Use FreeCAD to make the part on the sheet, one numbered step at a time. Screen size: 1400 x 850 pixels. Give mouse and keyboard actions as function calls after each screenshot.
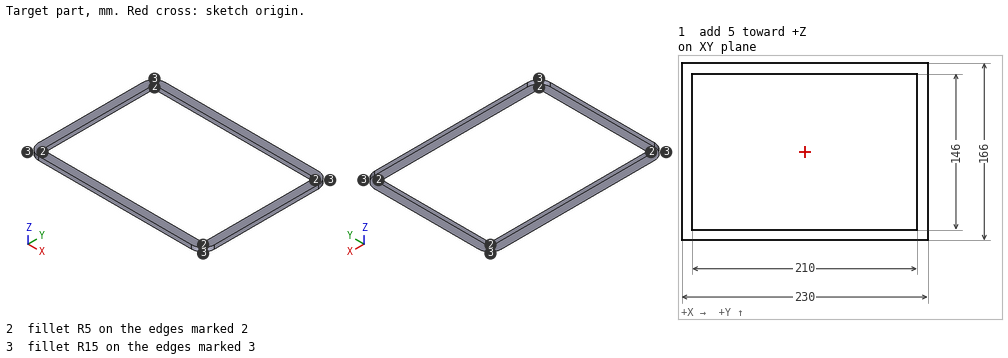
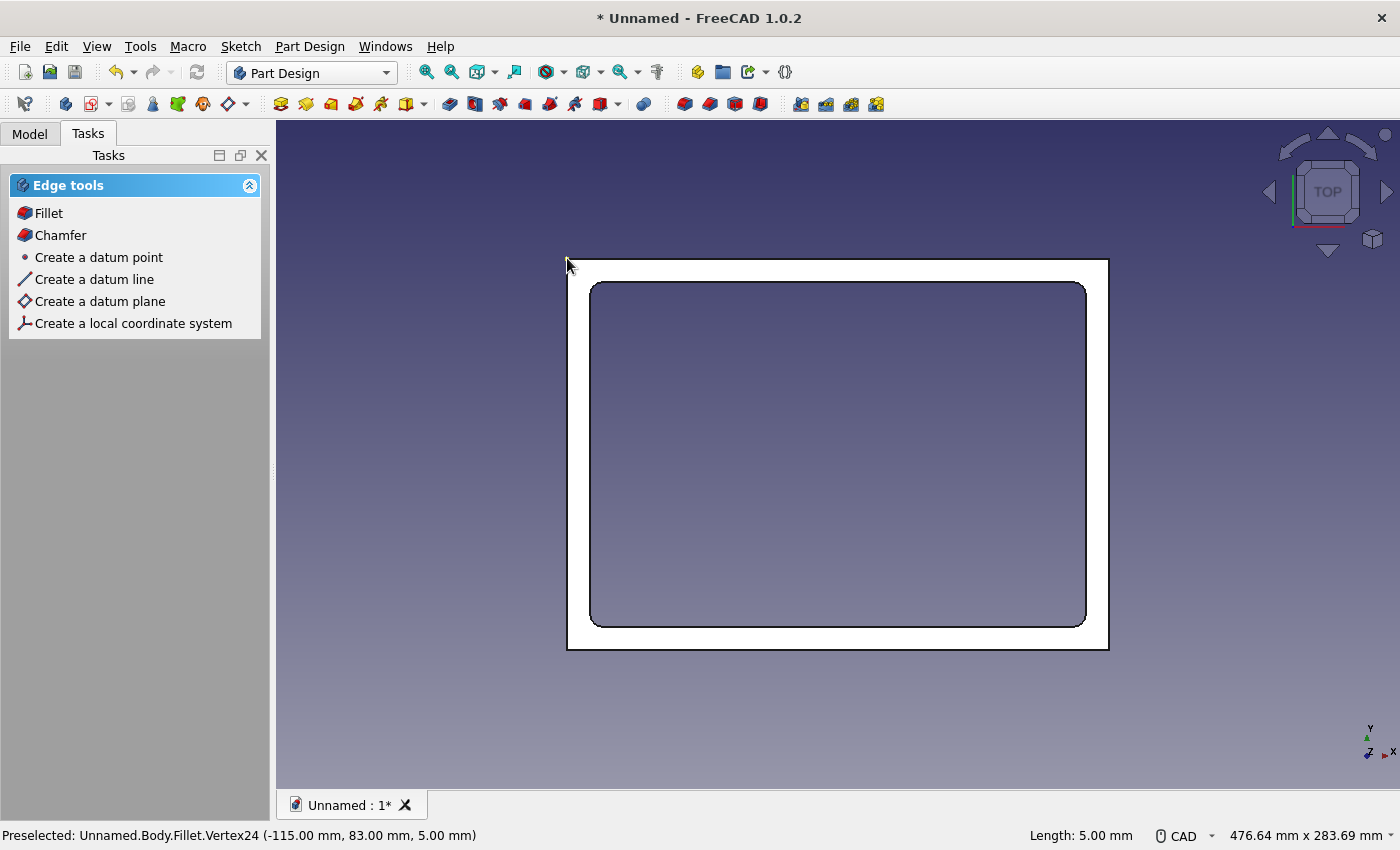
key(0)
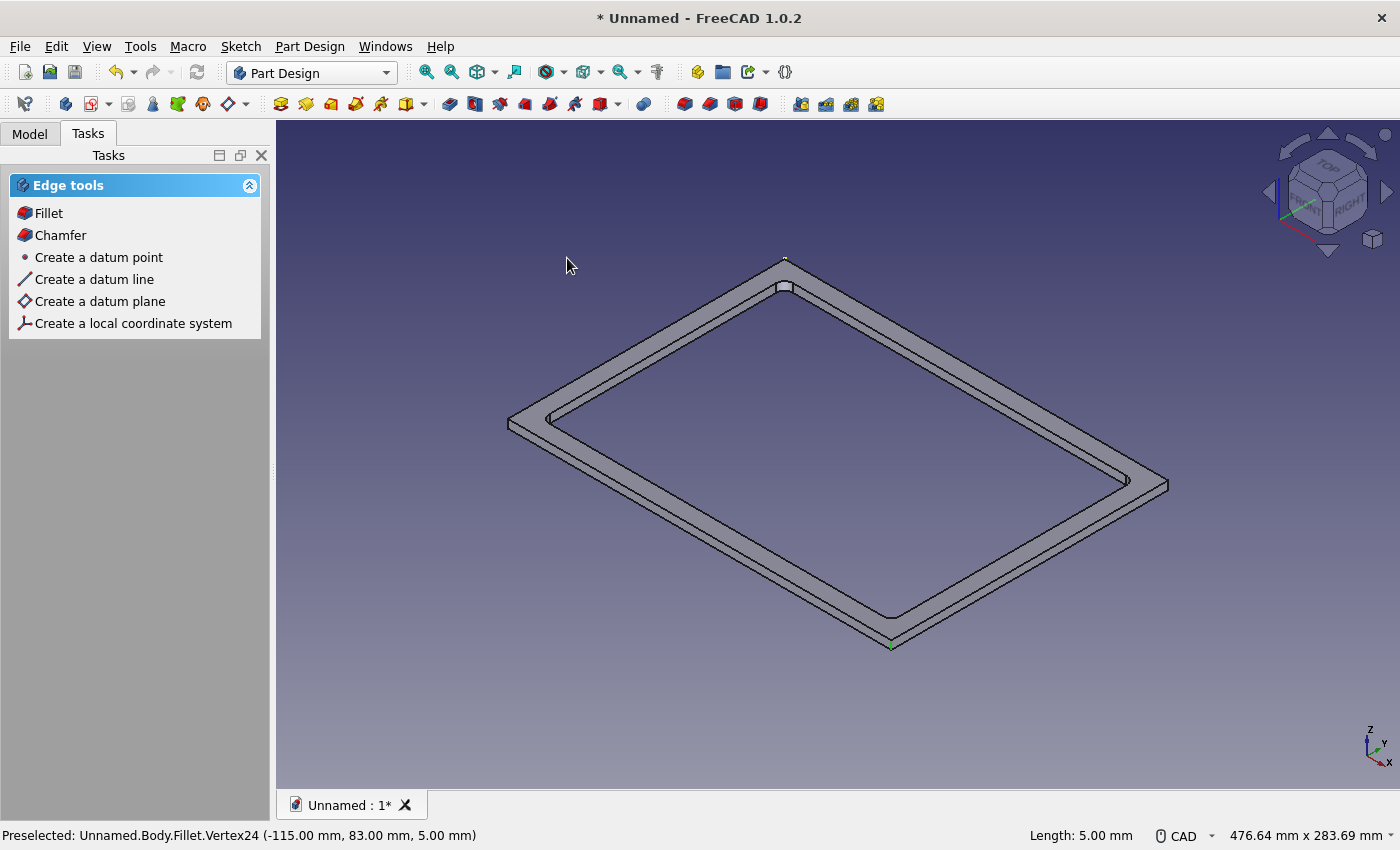
scroll(785, 263, up, 7)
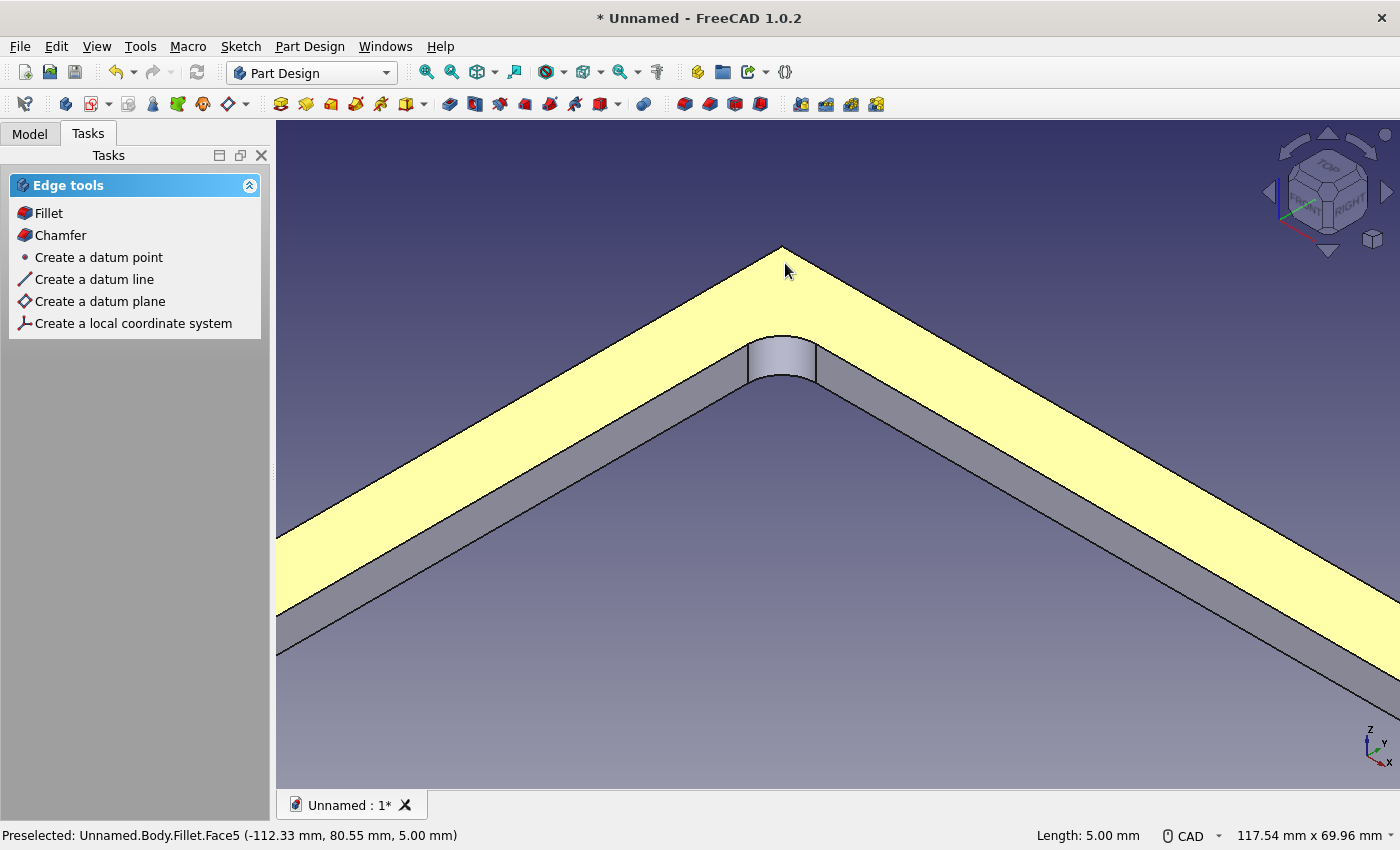
key(v)
key(f)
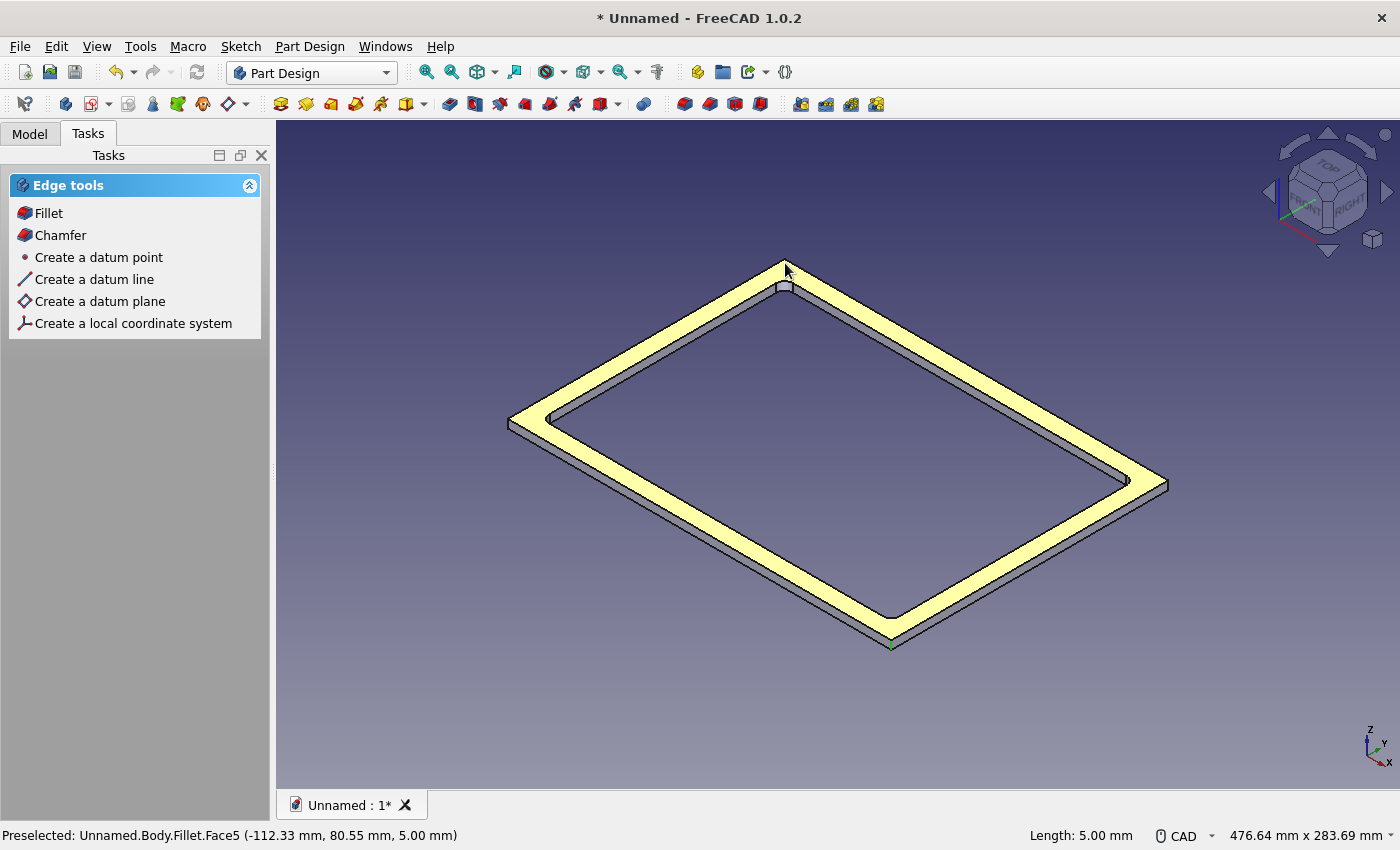
key(1)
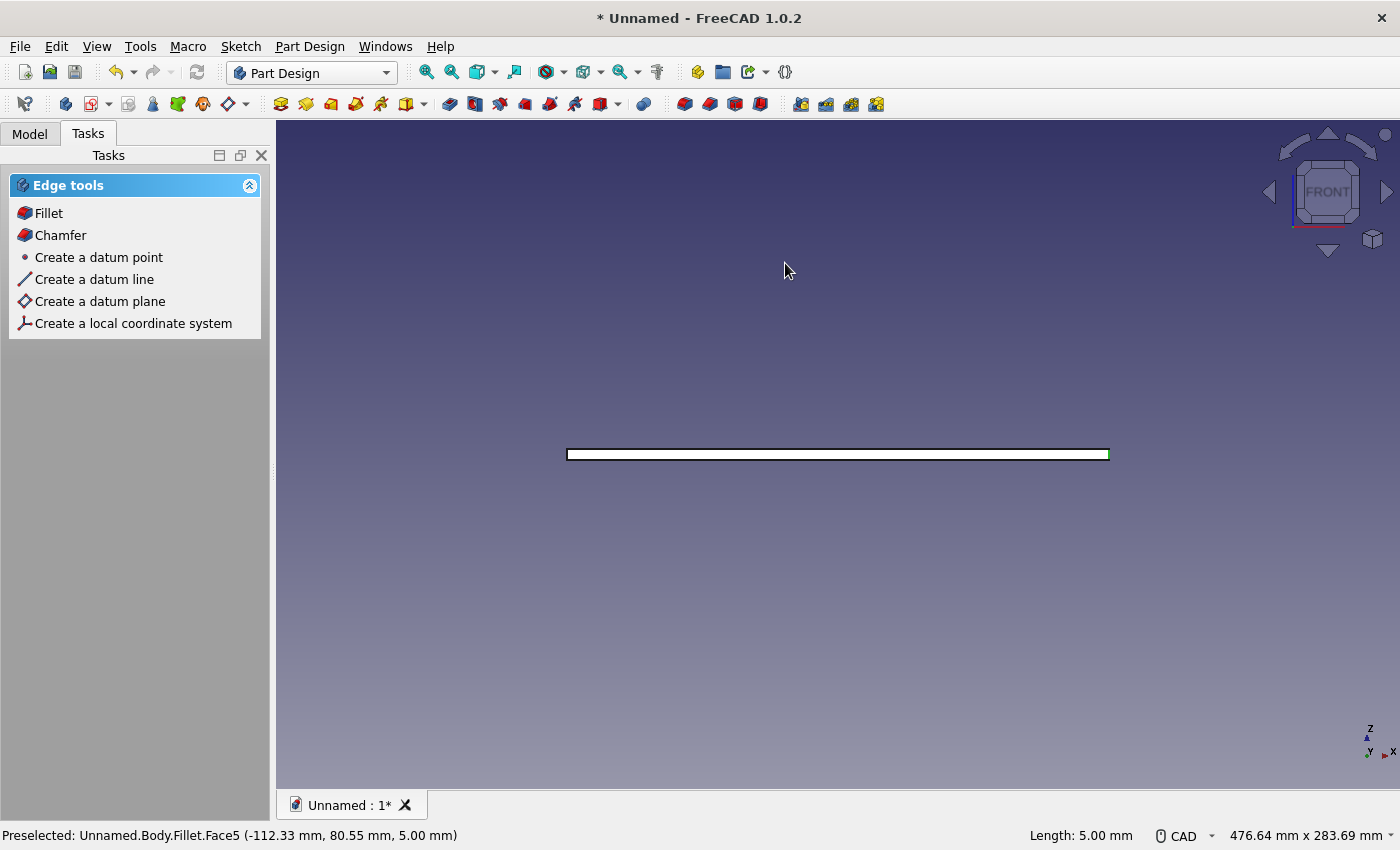
scroll(567, 453, up, 7)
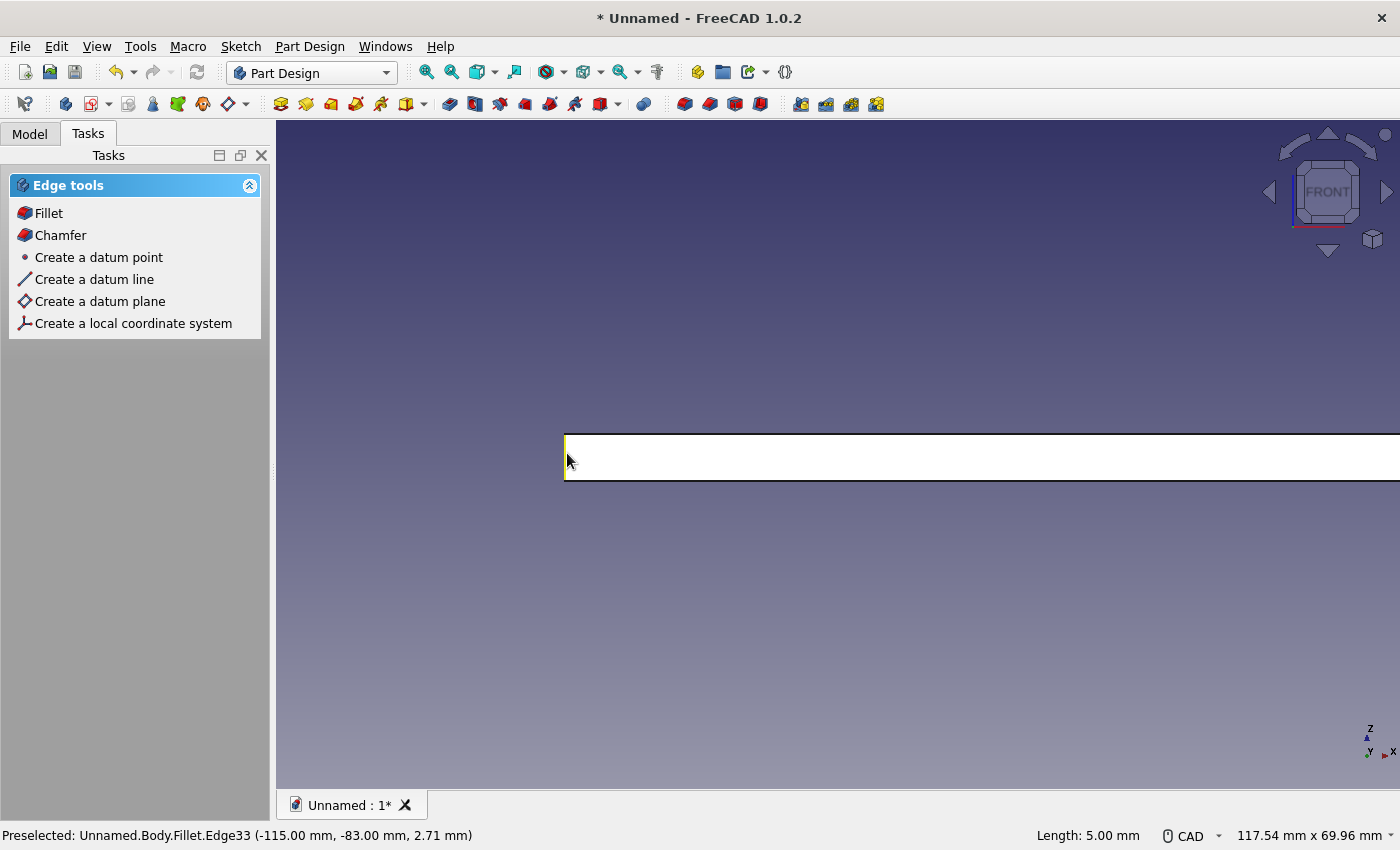
click(565, 457, ctrl)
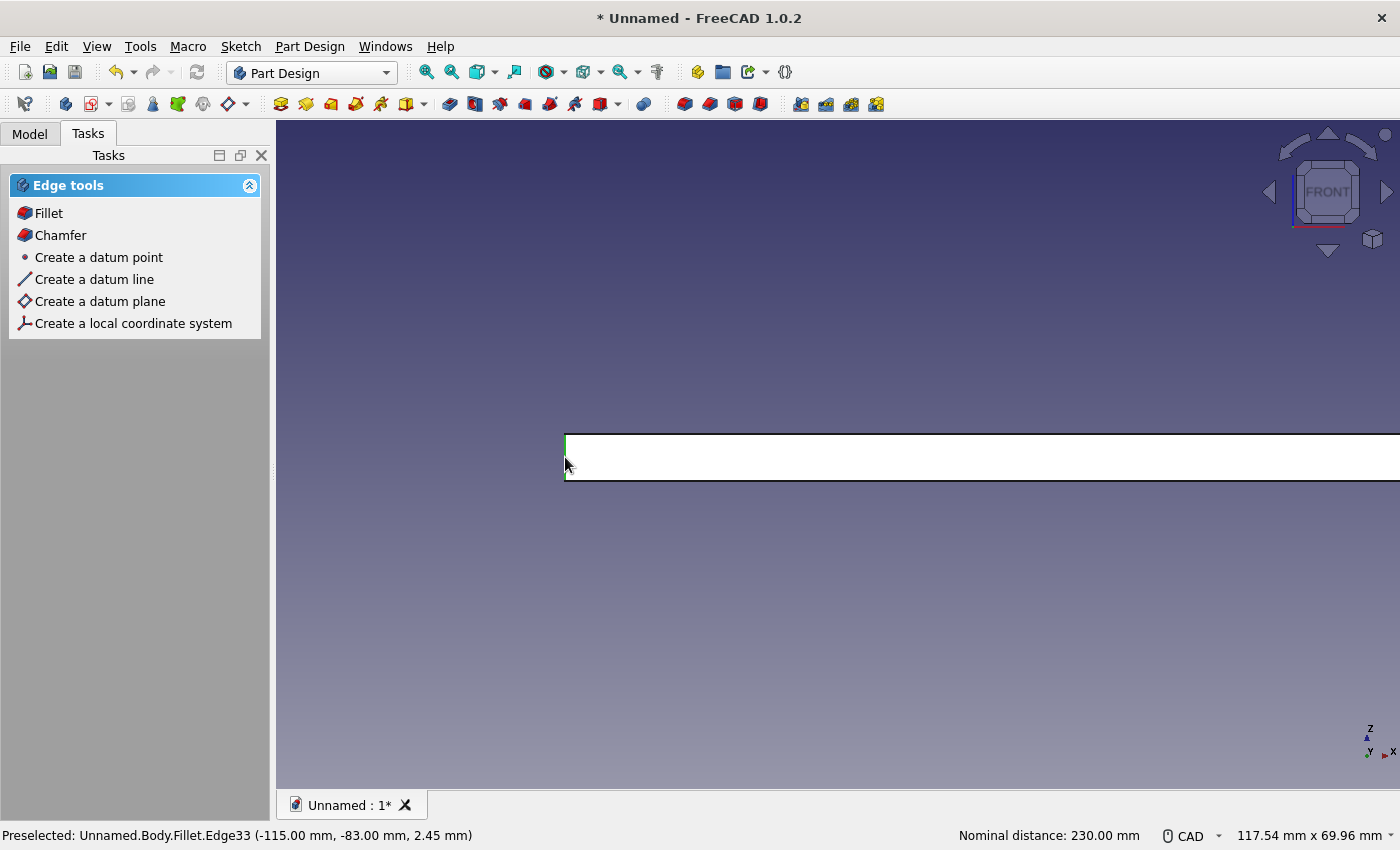
key(v)
key(f)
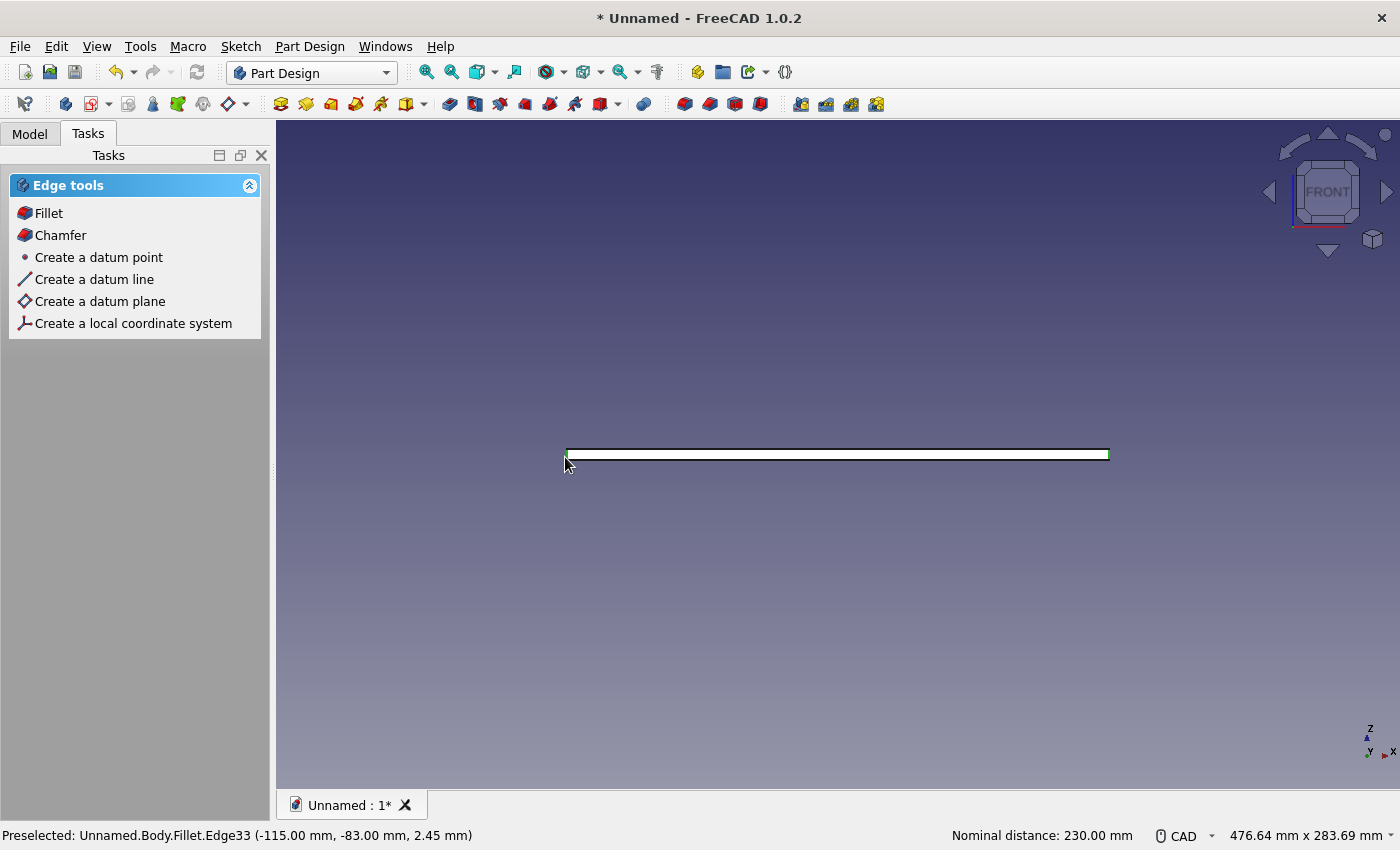
key(3)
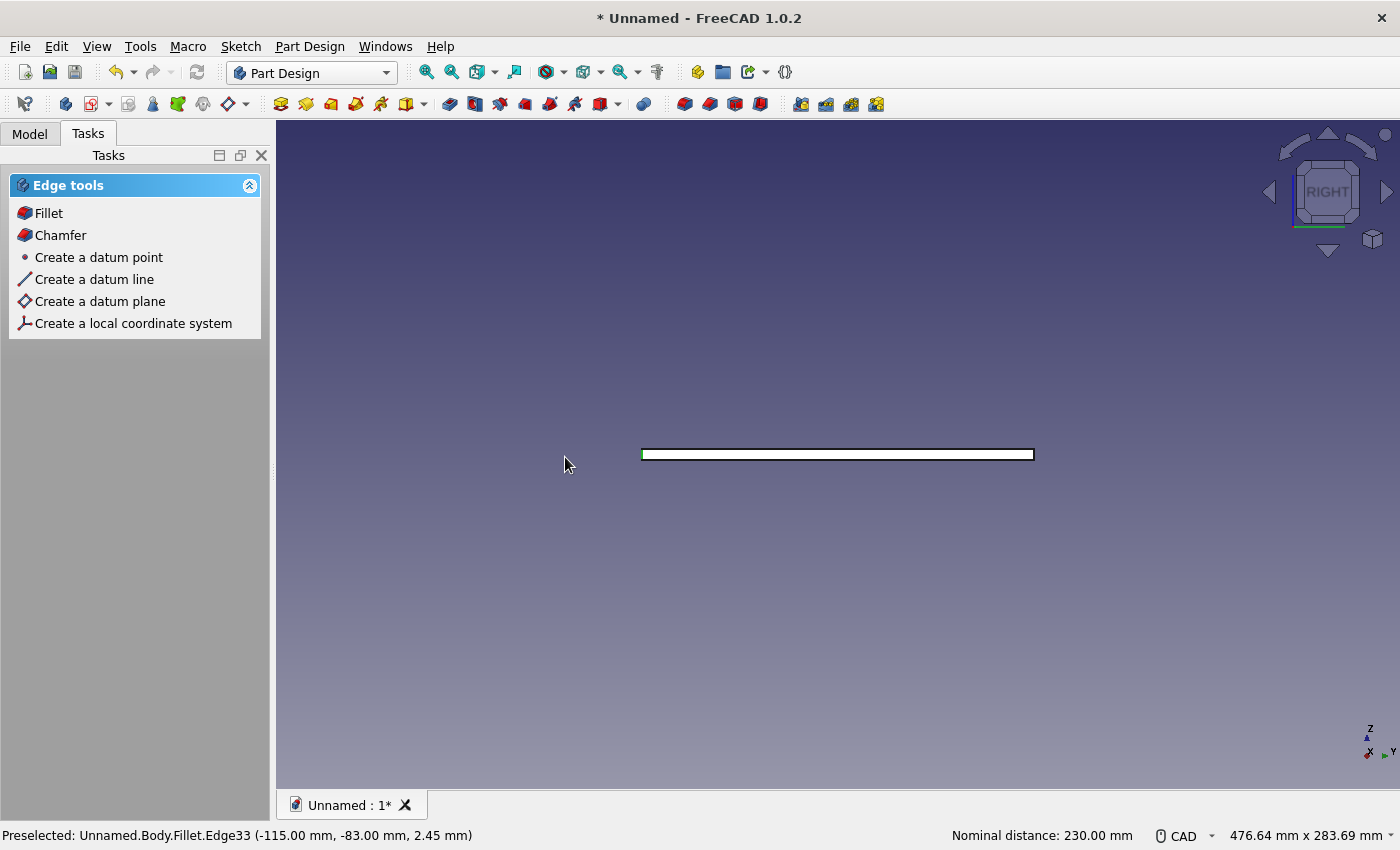
key(v)
key(f)